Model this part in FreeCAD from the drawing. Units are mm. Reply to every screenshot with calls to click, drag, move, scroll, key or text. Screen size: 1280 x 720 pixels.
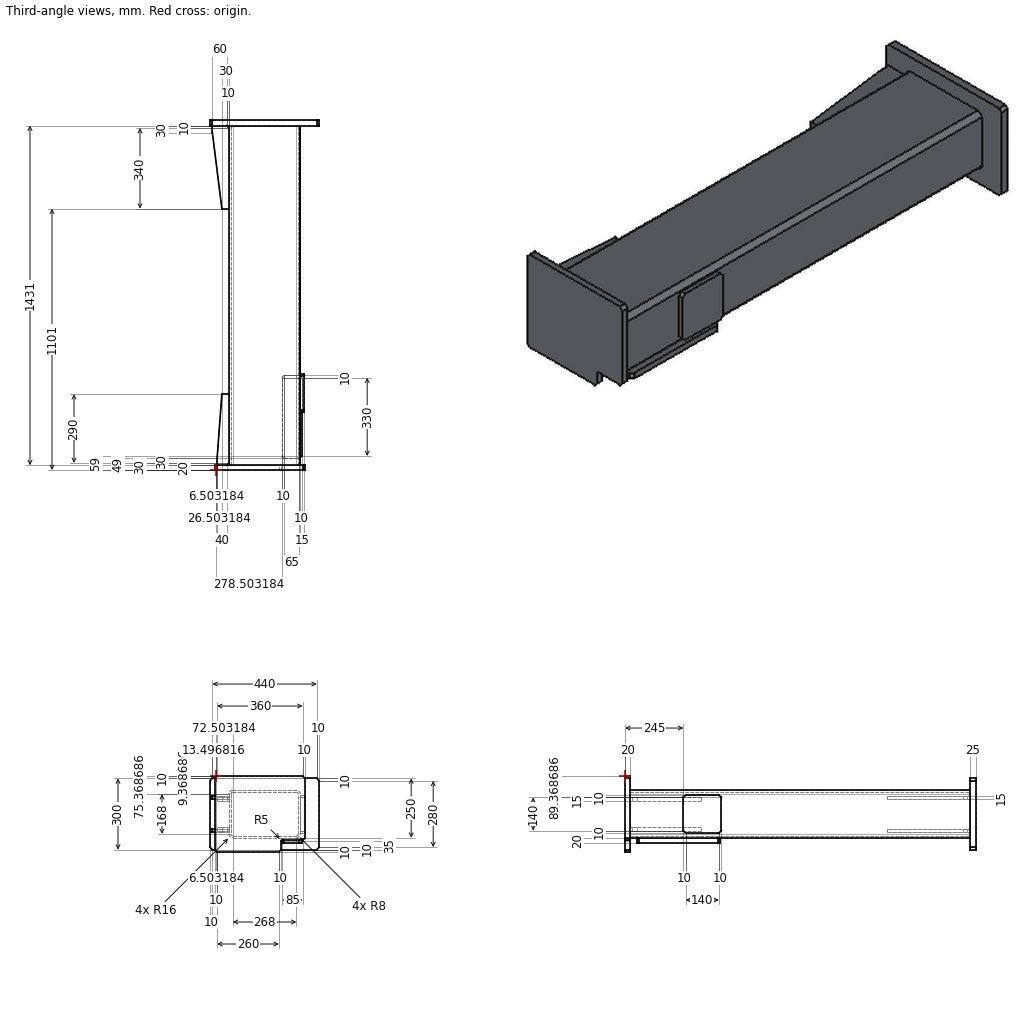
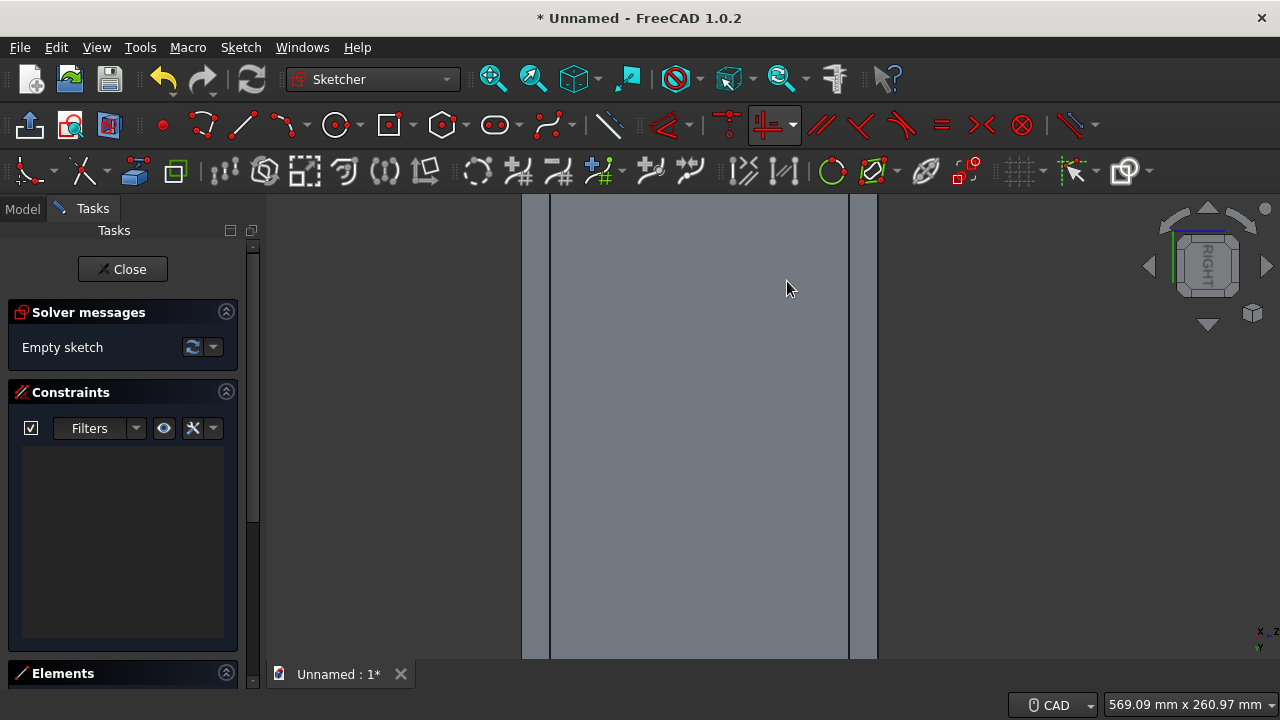
click(204, 126)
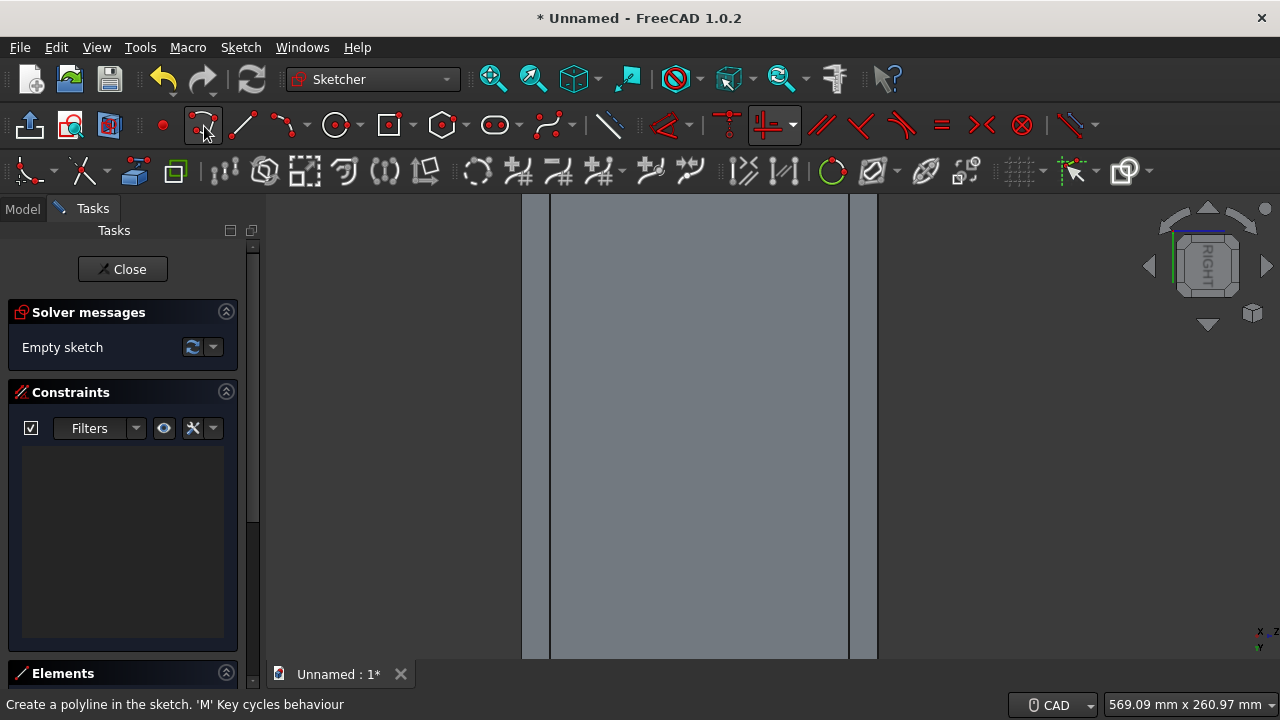
click(824, 282)
click(575, 282)
click(557, 300)
click(557, 549)
click(575, 567)
click(824, 567)
click(842, 549)
click(842, 300)
click(824, 283)
key(Escape)
key(Escape)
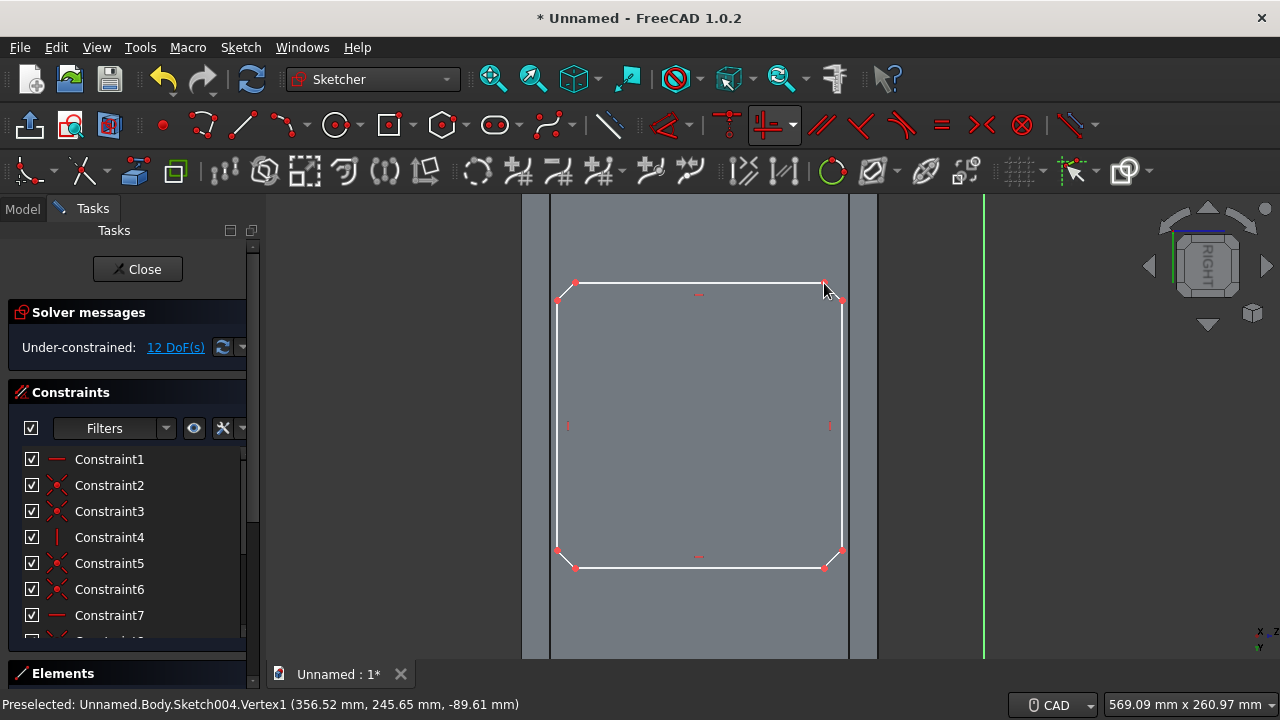
click(664, 126)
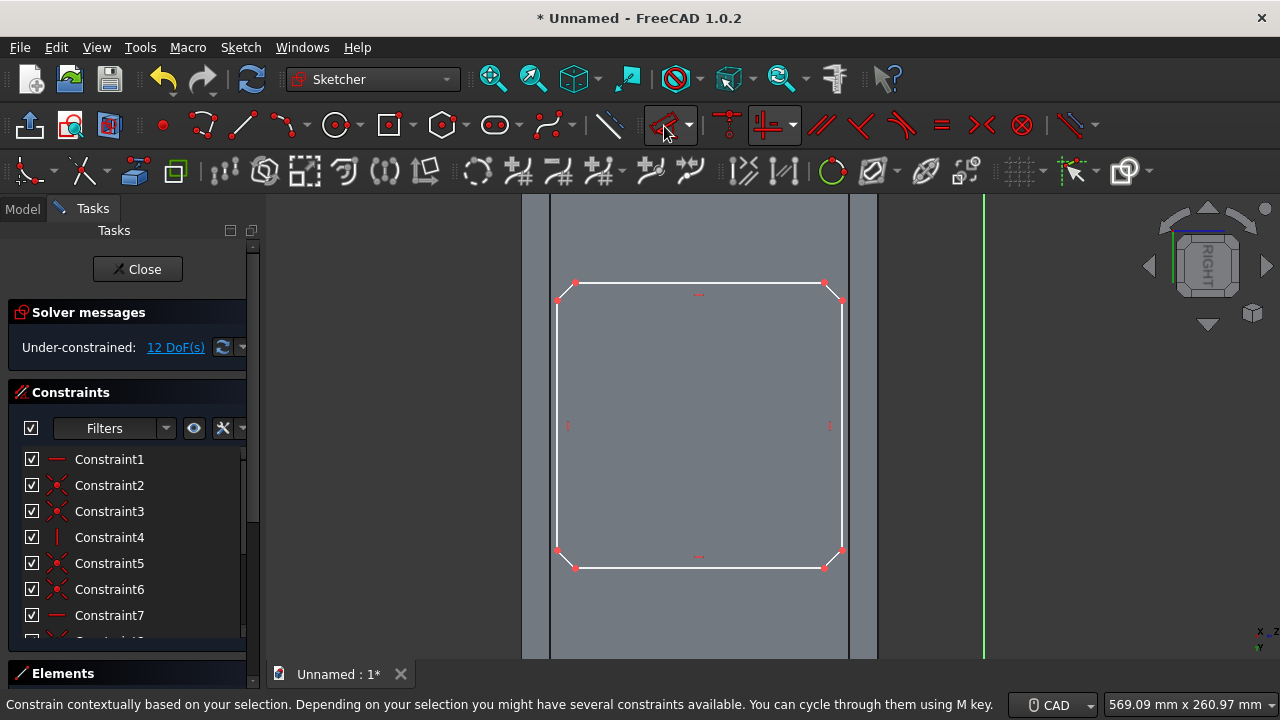
click(749, 283)
click(699, 249)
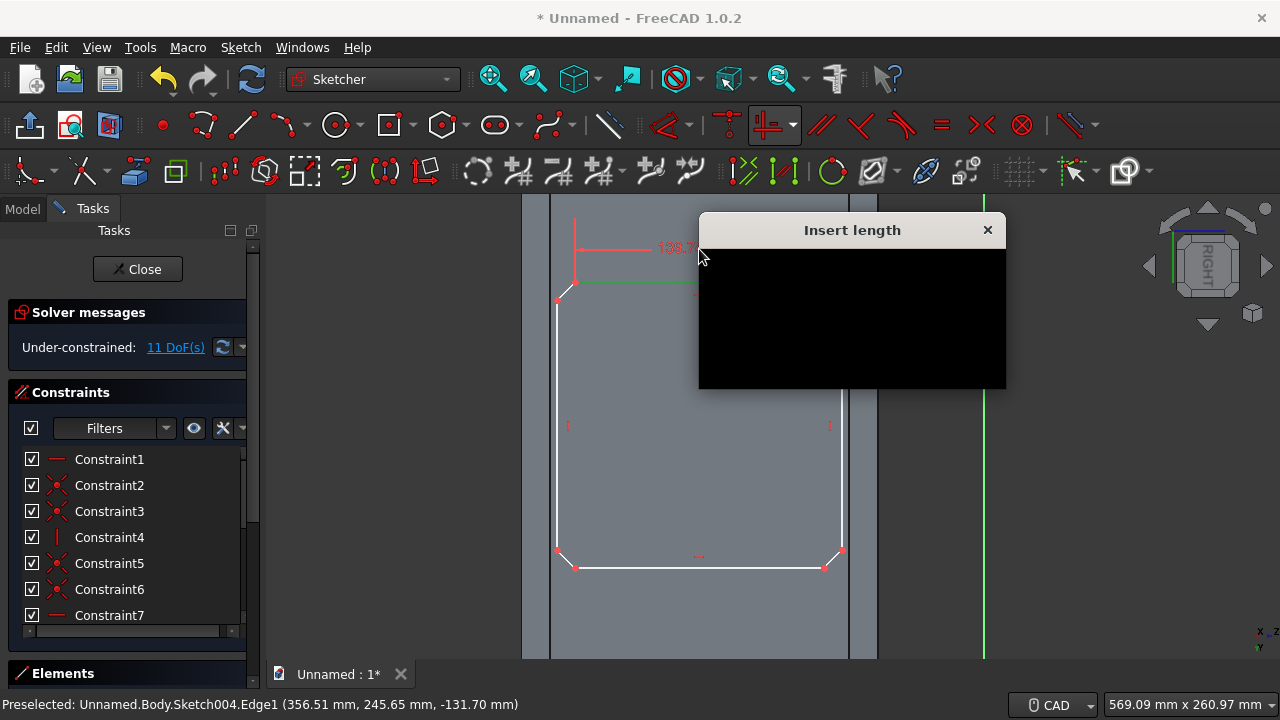
text(140)
key(Return)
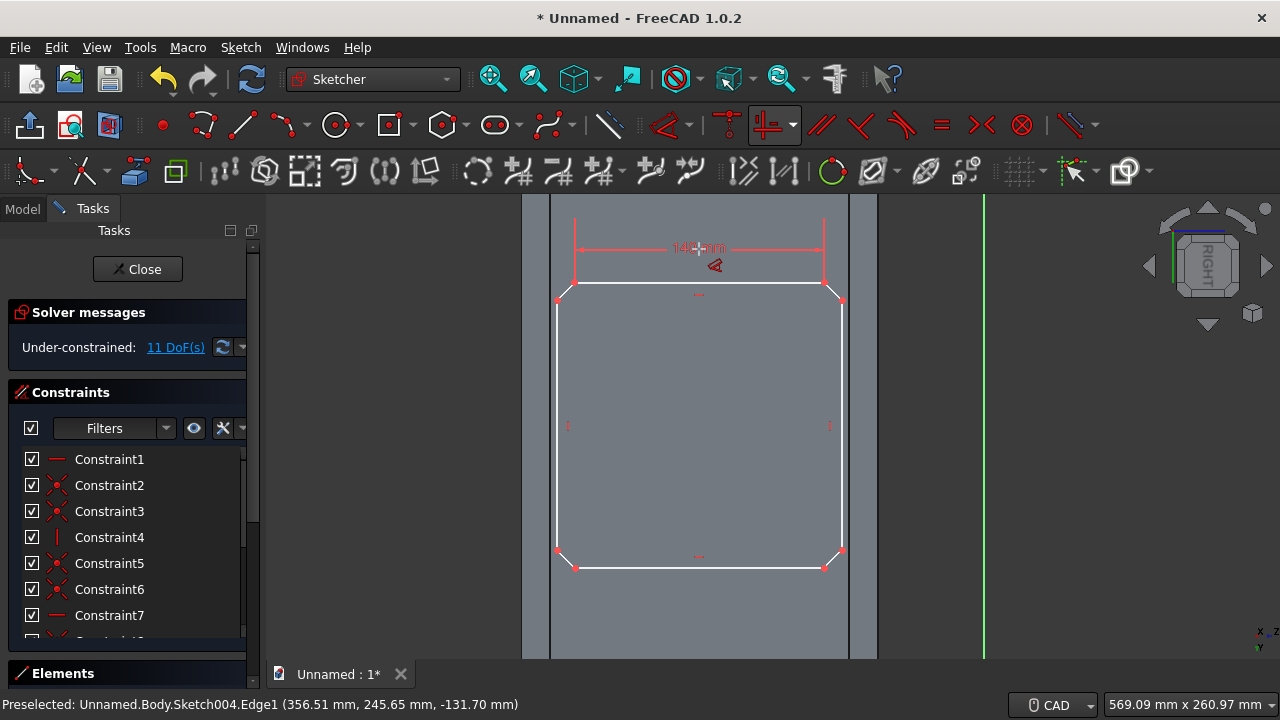
click(557, 376)
click(523, 426)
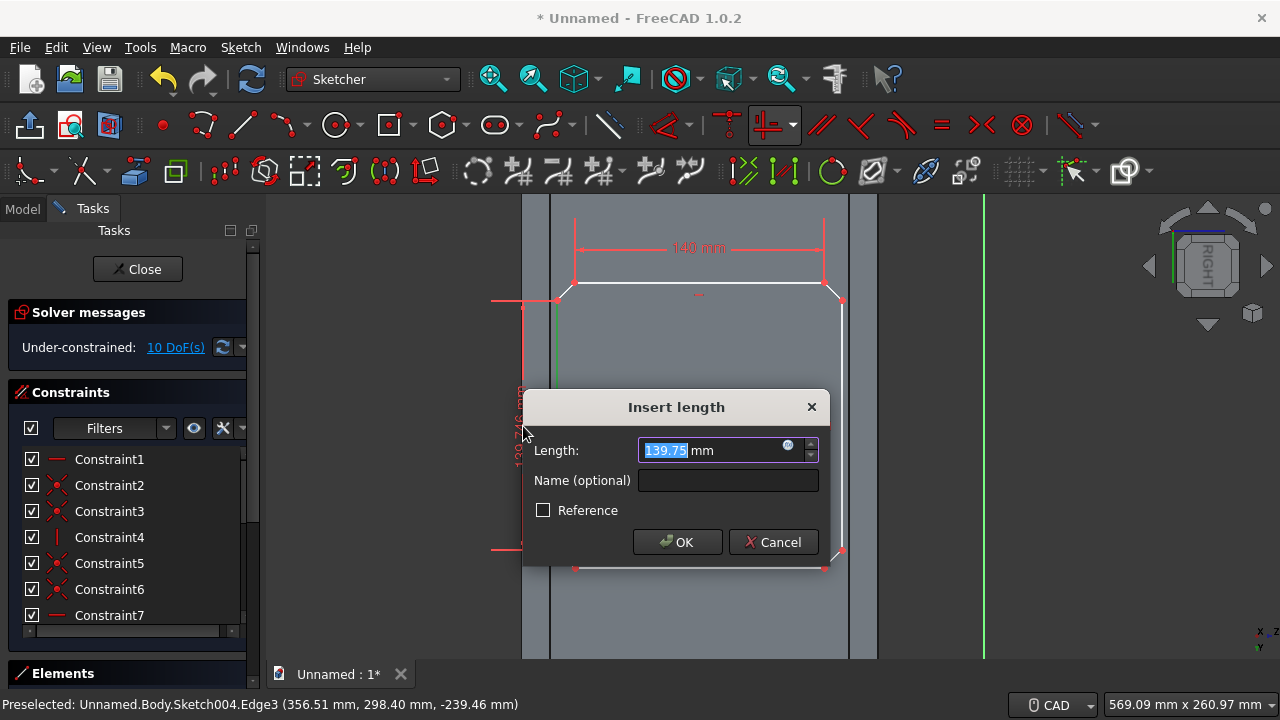
text(140)
key(Return)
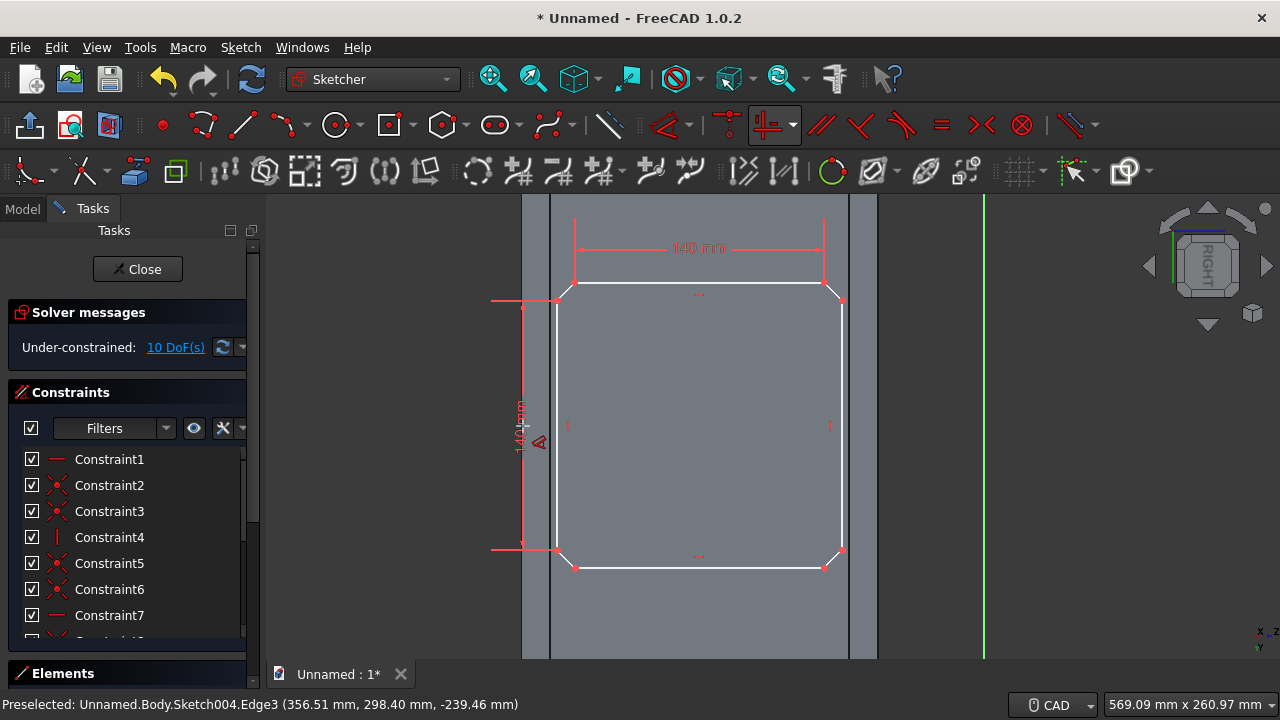
click(650, 568)
click(699, 602)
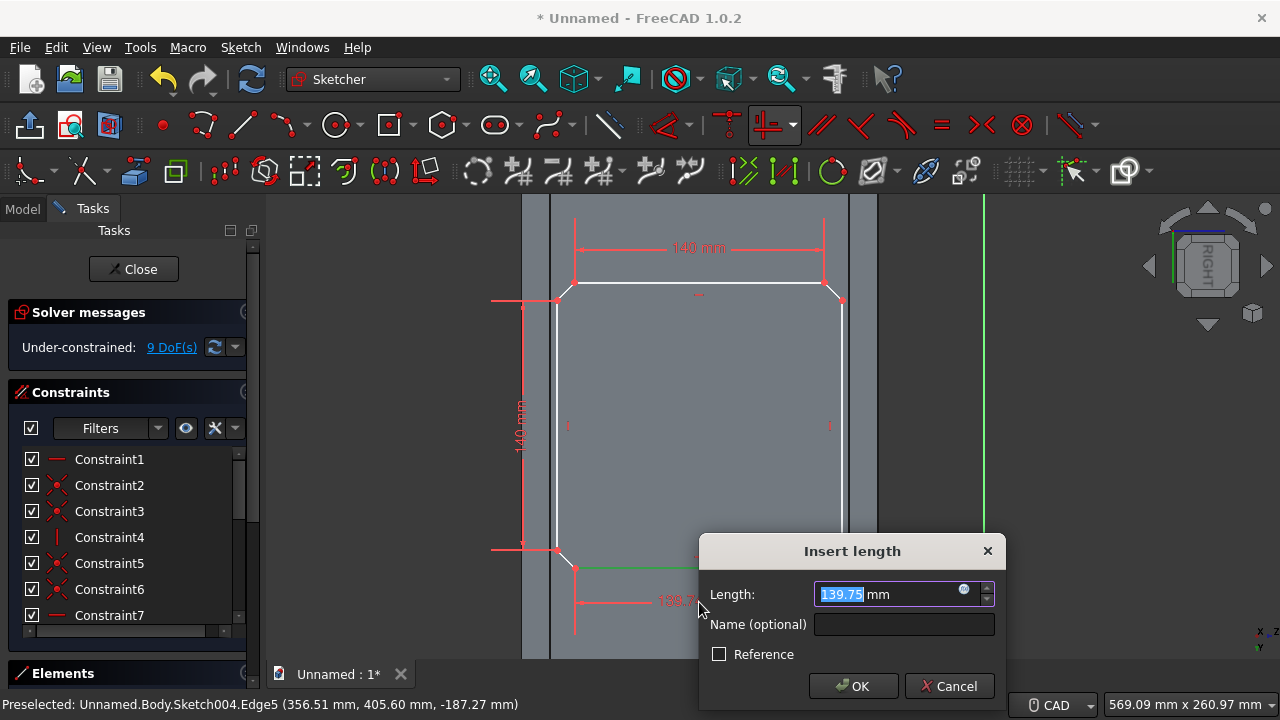
text(140)
key(Return)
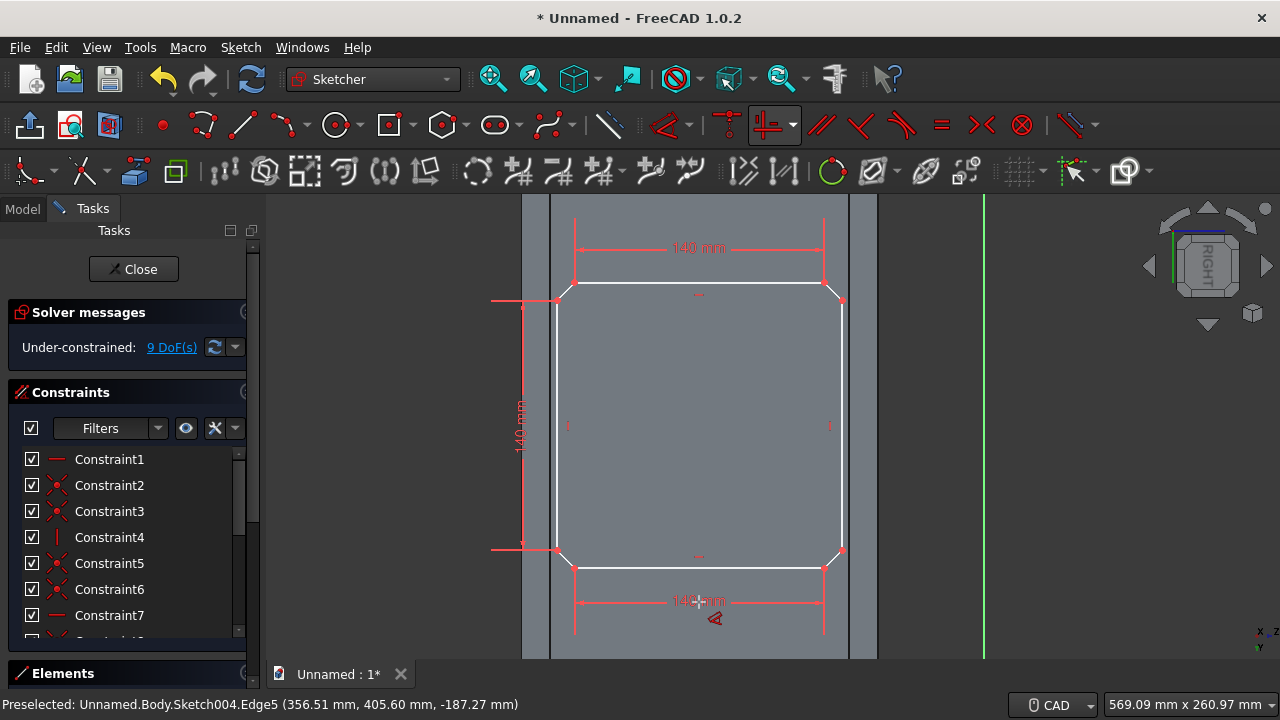
click(842, 475)
click(876, 426)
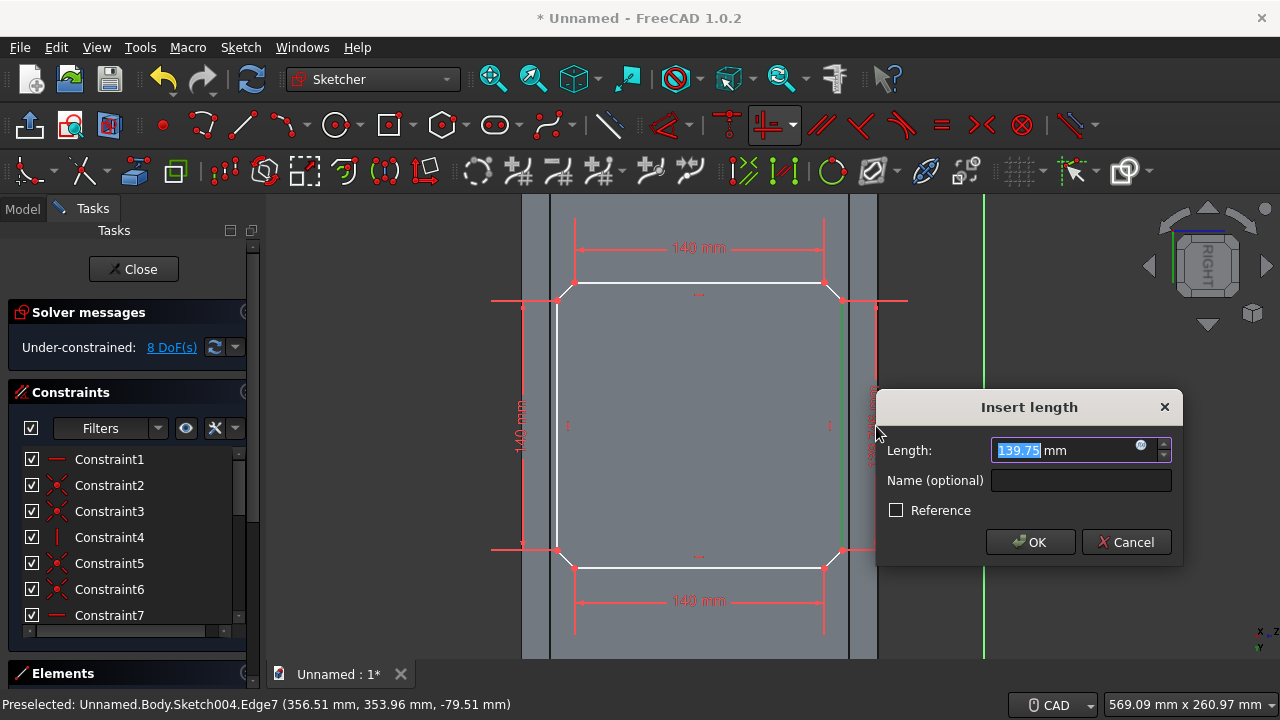
text(140)
key(Return)